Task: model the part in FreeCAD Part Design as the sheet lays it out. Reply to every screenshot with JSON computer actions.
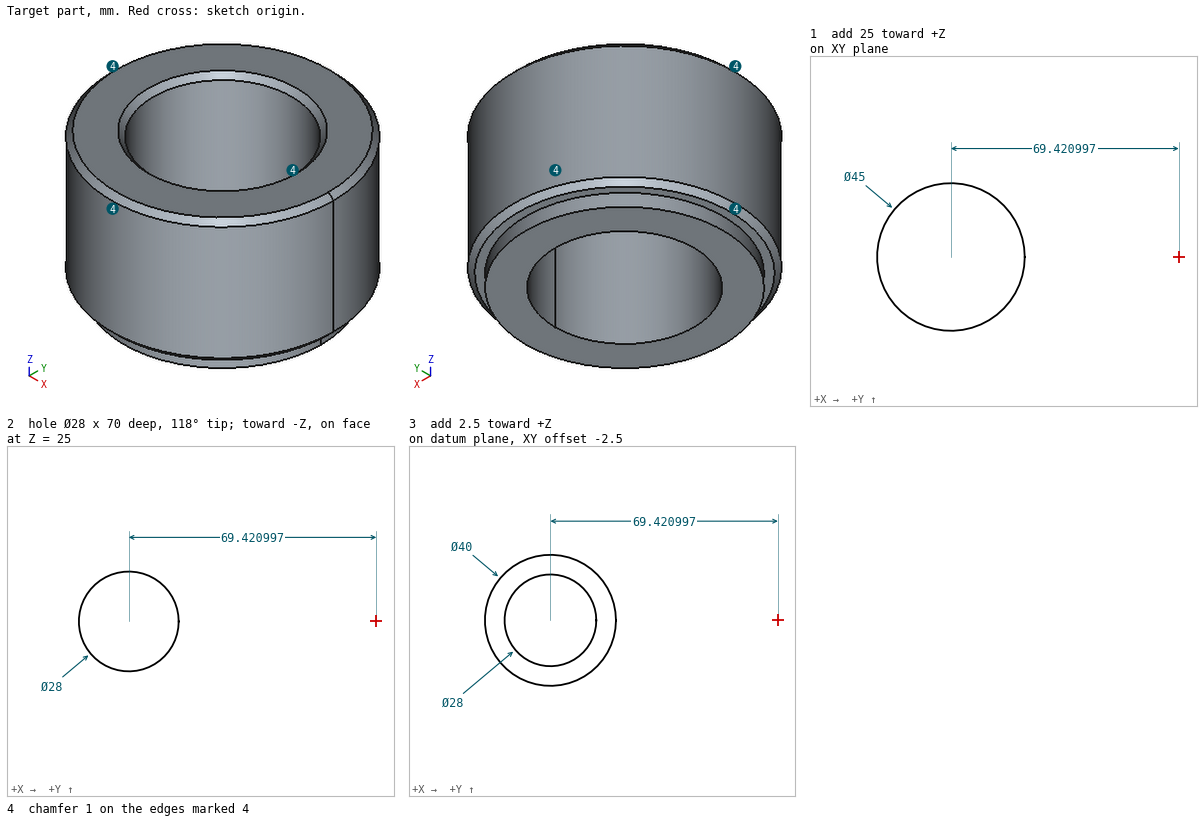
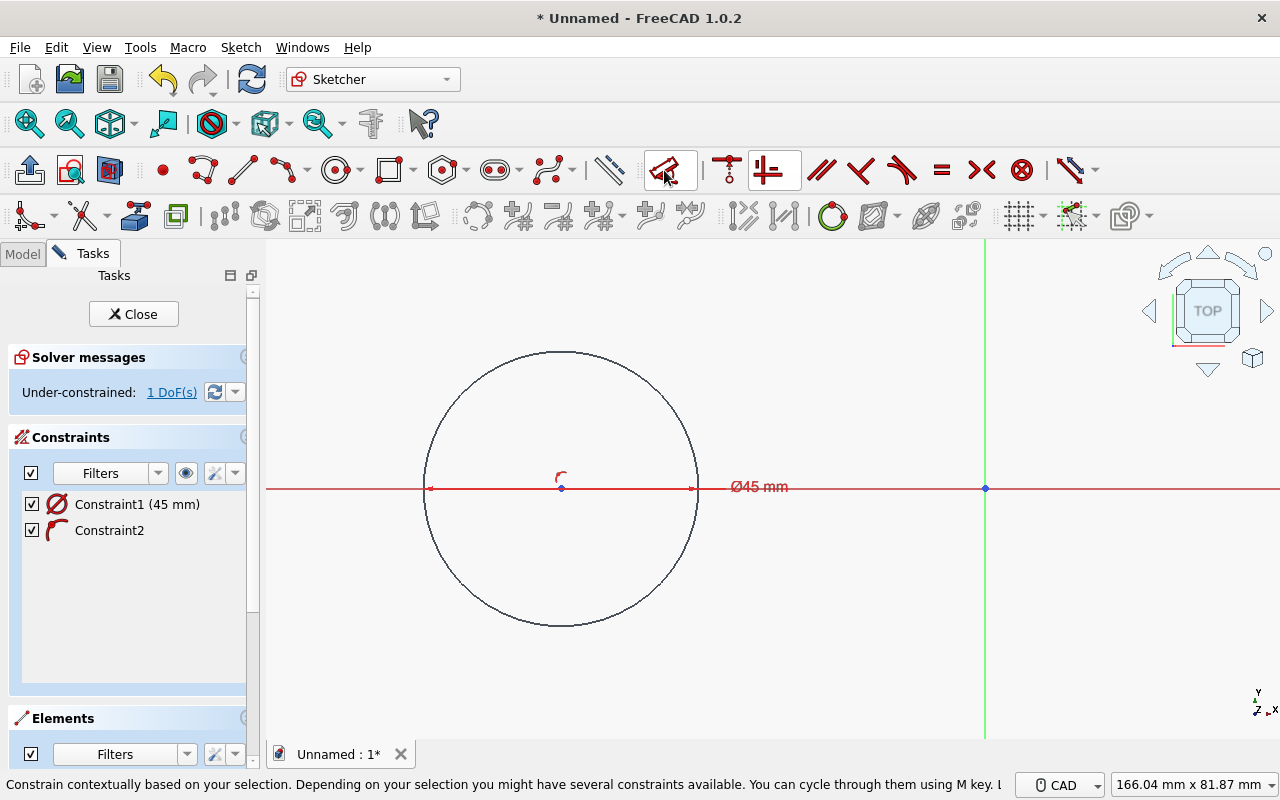
{"action": "left_click", "coordinate": [561, 489]}
{"action": "left_click", "coordinate": [773, 523]}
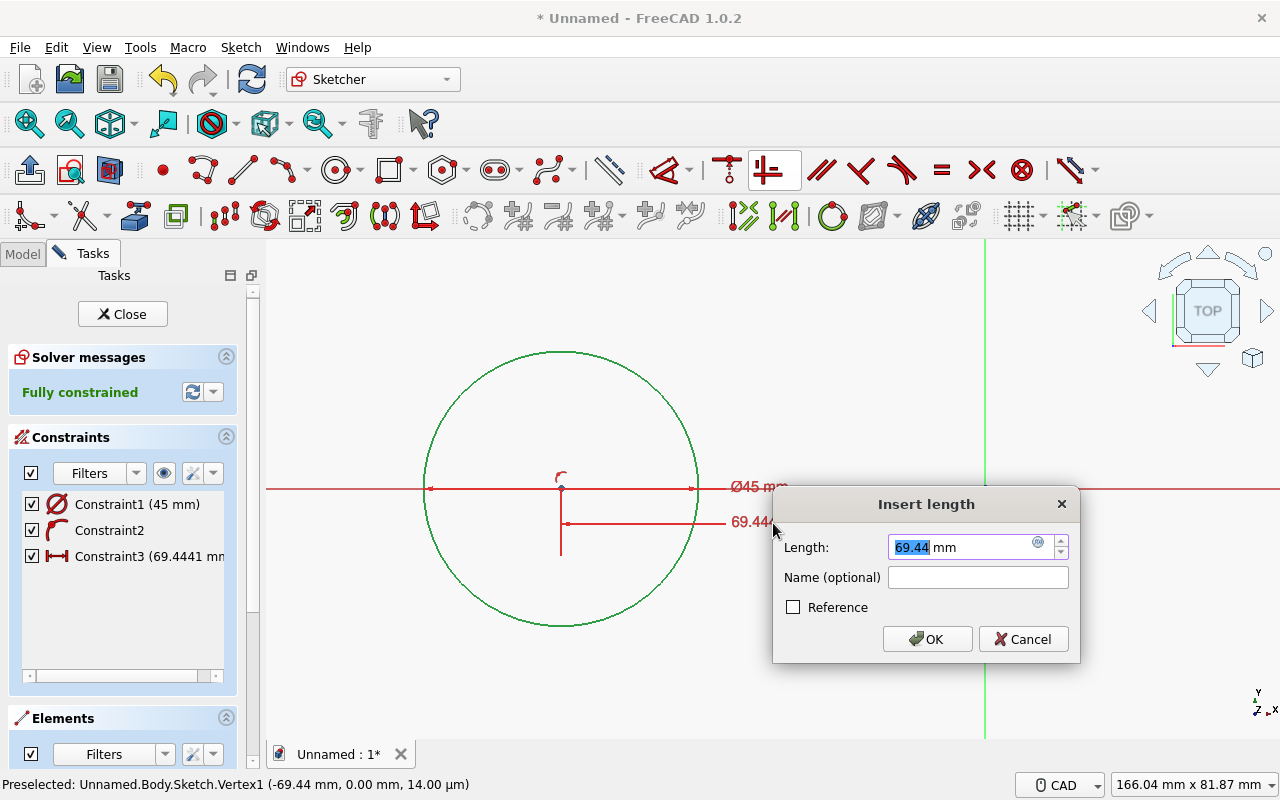
{"action": "type", "text": "69.420997"}
{"action": "key", "text": "Return"}
{"action": "key", "text": "Escape"}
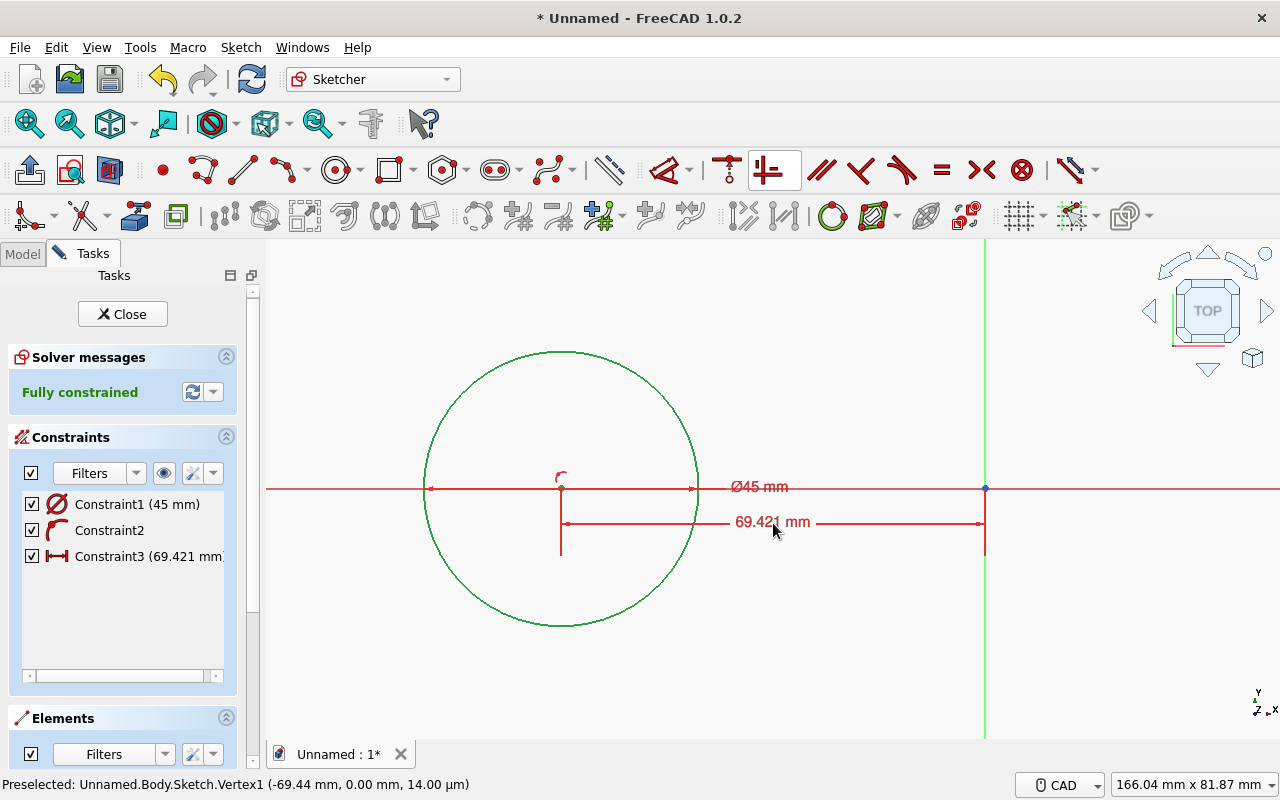
{"action": "left_click", "coordinate": [123, 314]}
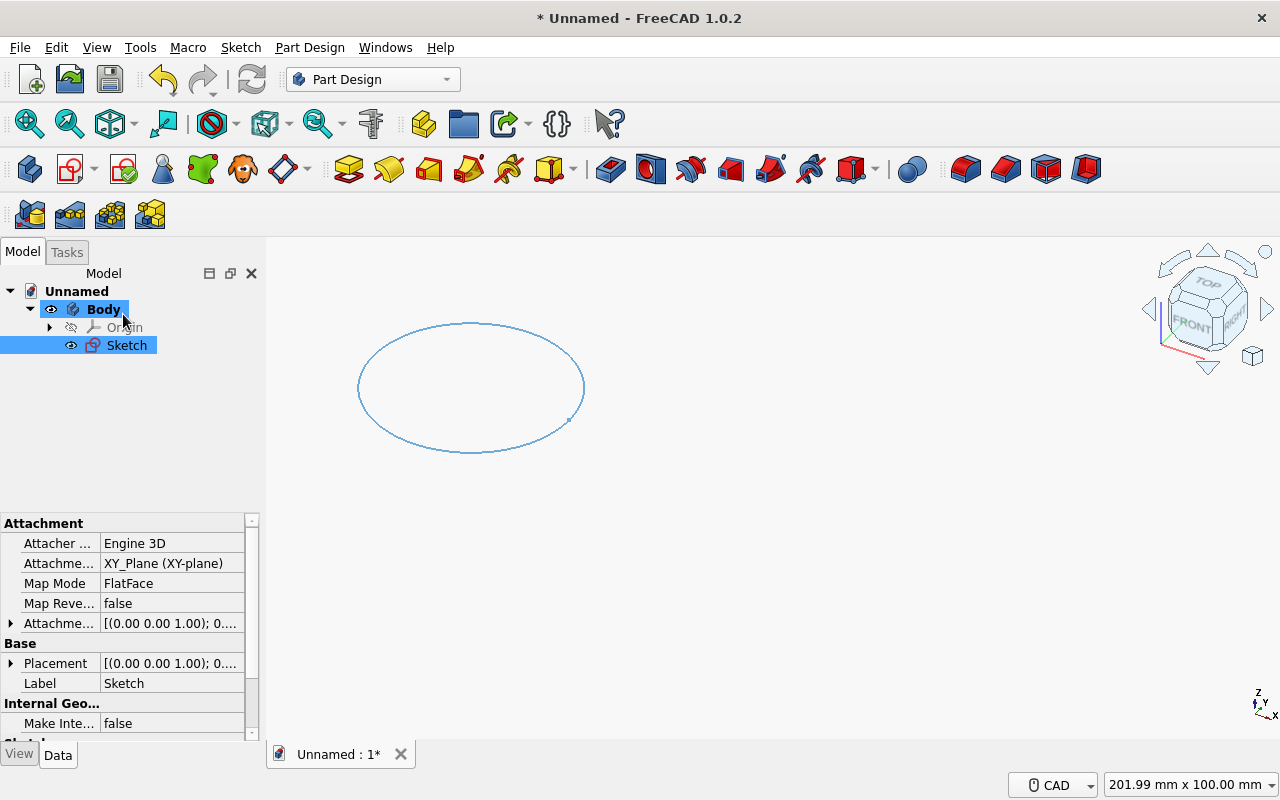
{"action": "left_click", "coordinate": [350, 170]}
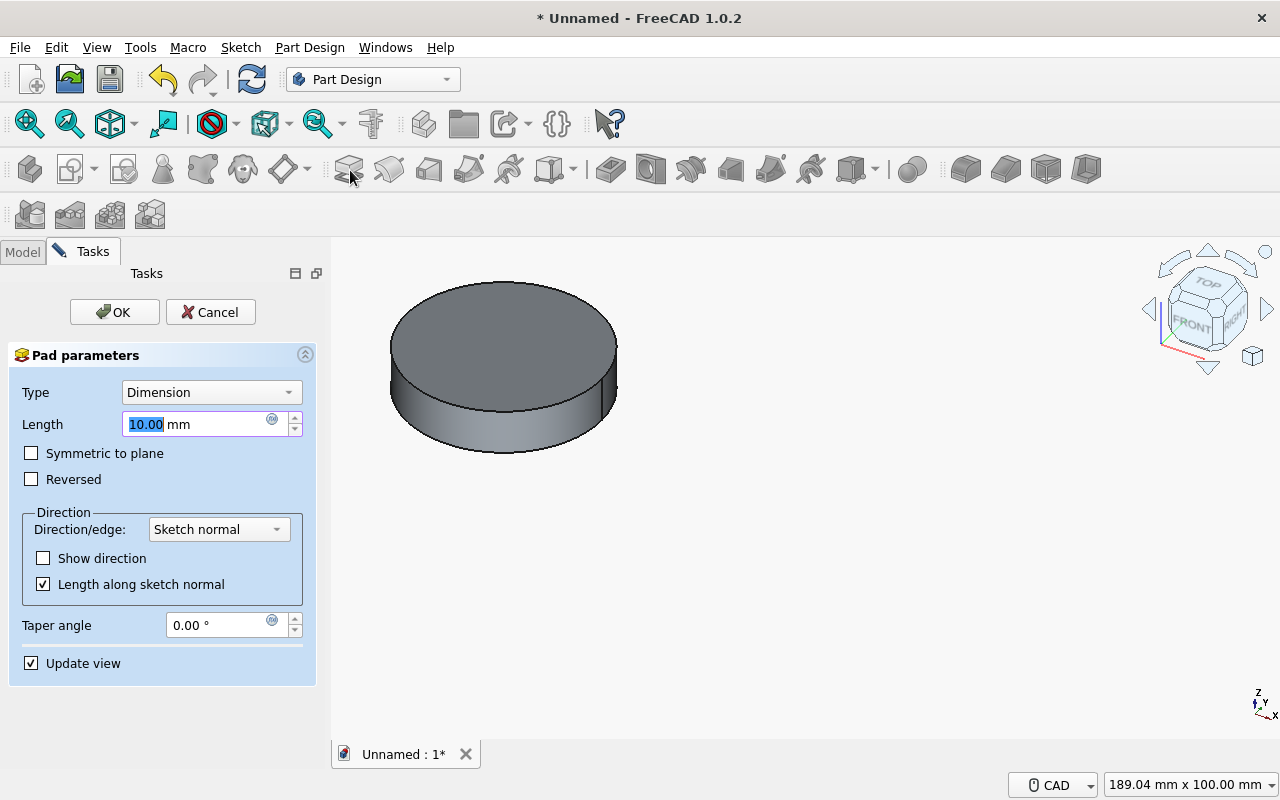
{"action": "type", "text": "25"}
{"action": "key", "text": "Tab"}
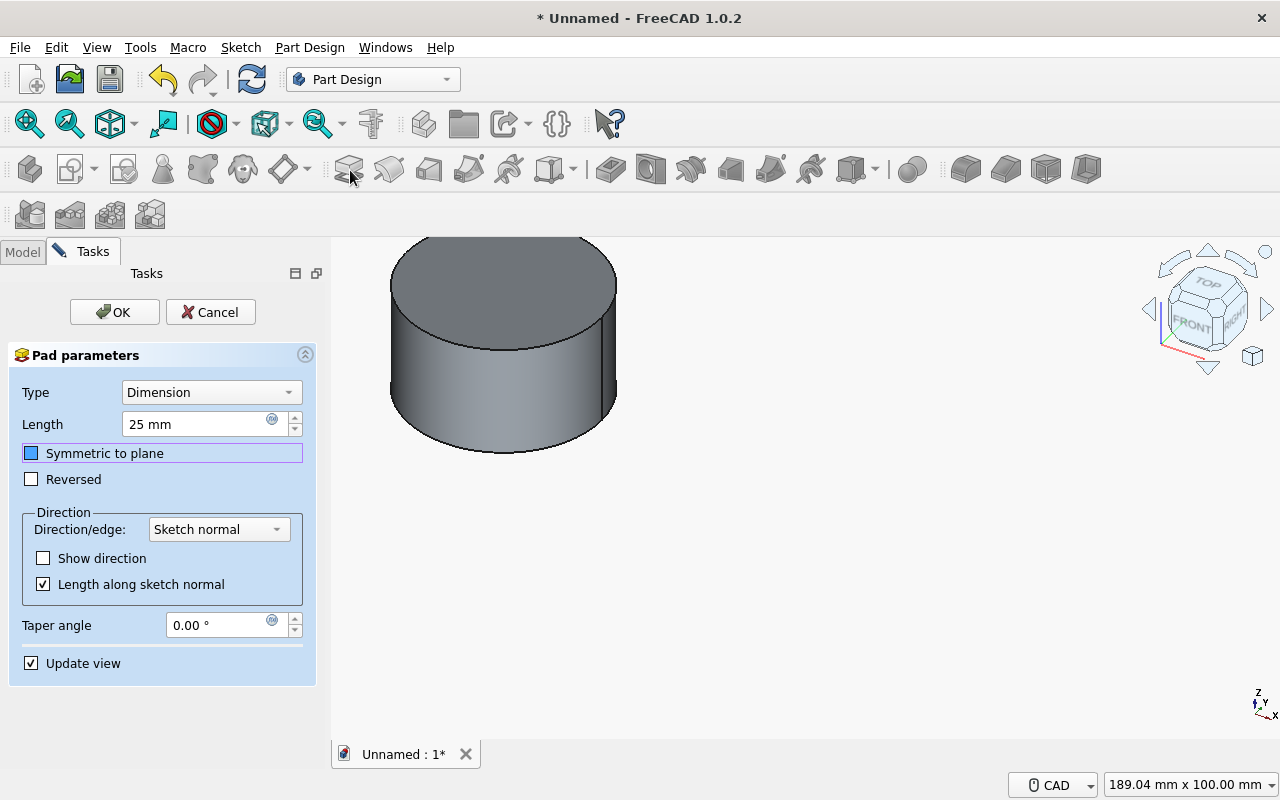
{"action": "left_click", "coordinate": [115, 312]}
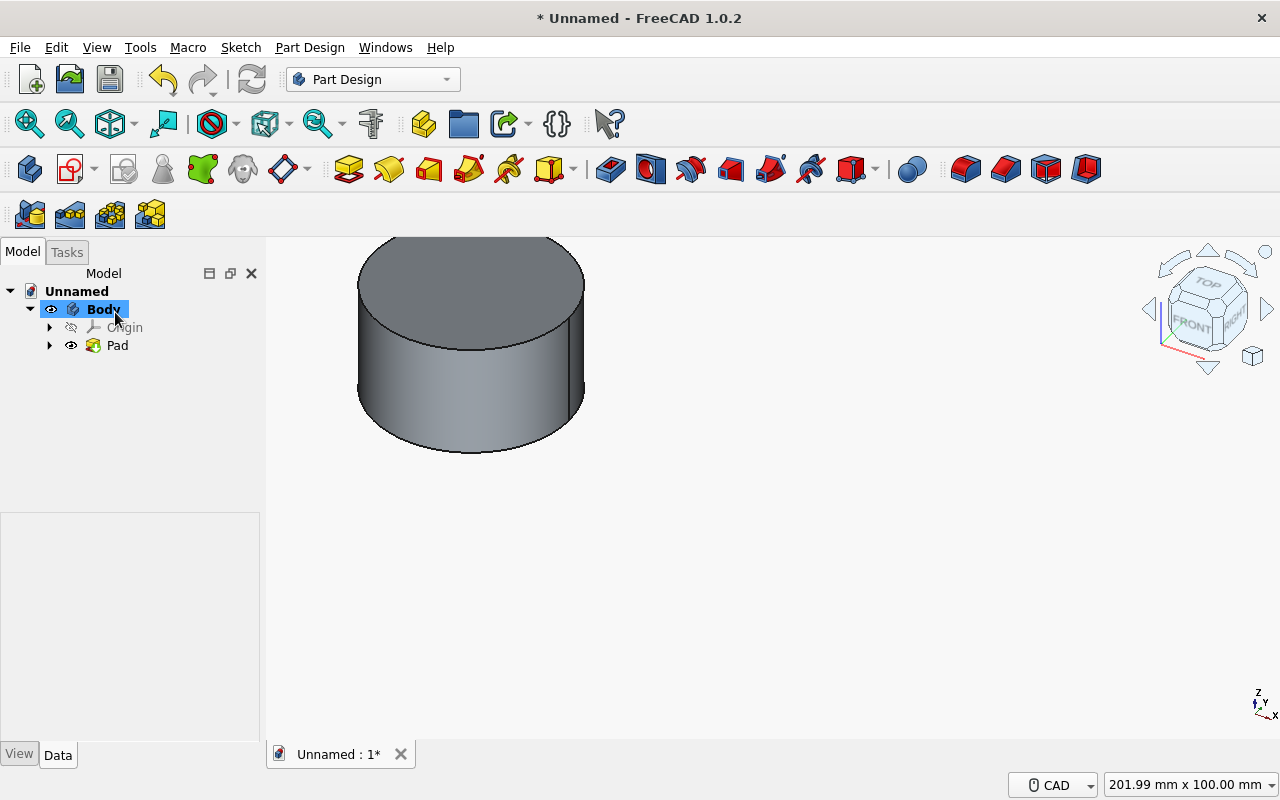
{"action": "key", "text": "v f"}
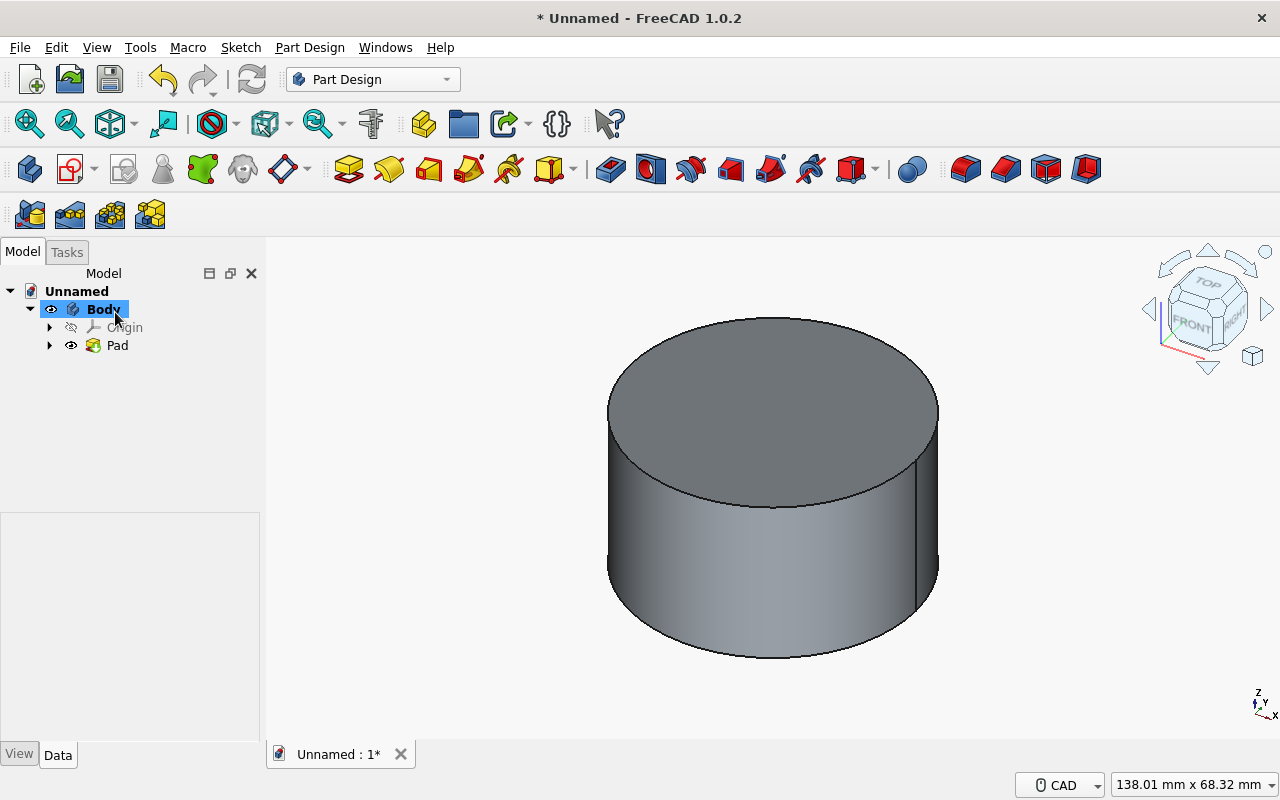
{"action": "left_click", "coordinate": [773, 412]}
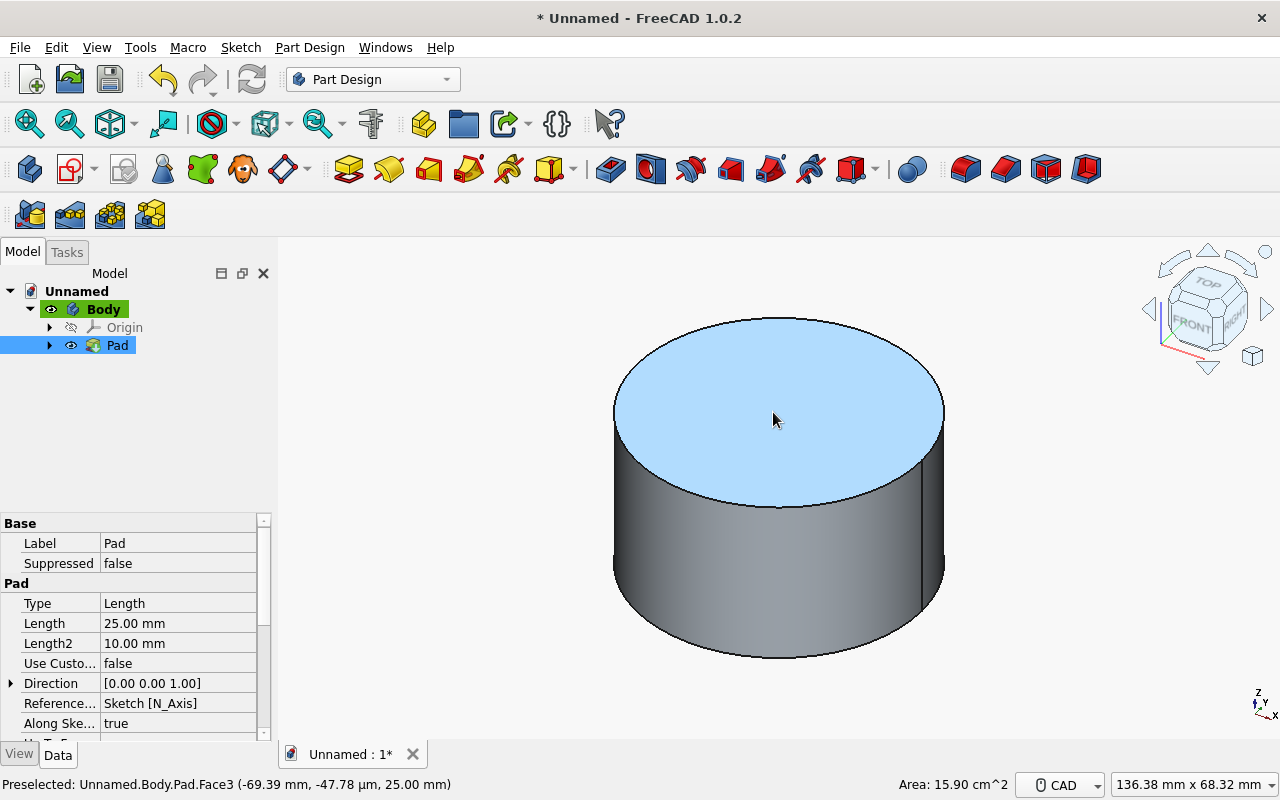
{"action": "left_click", "coordinate": [70, 170]}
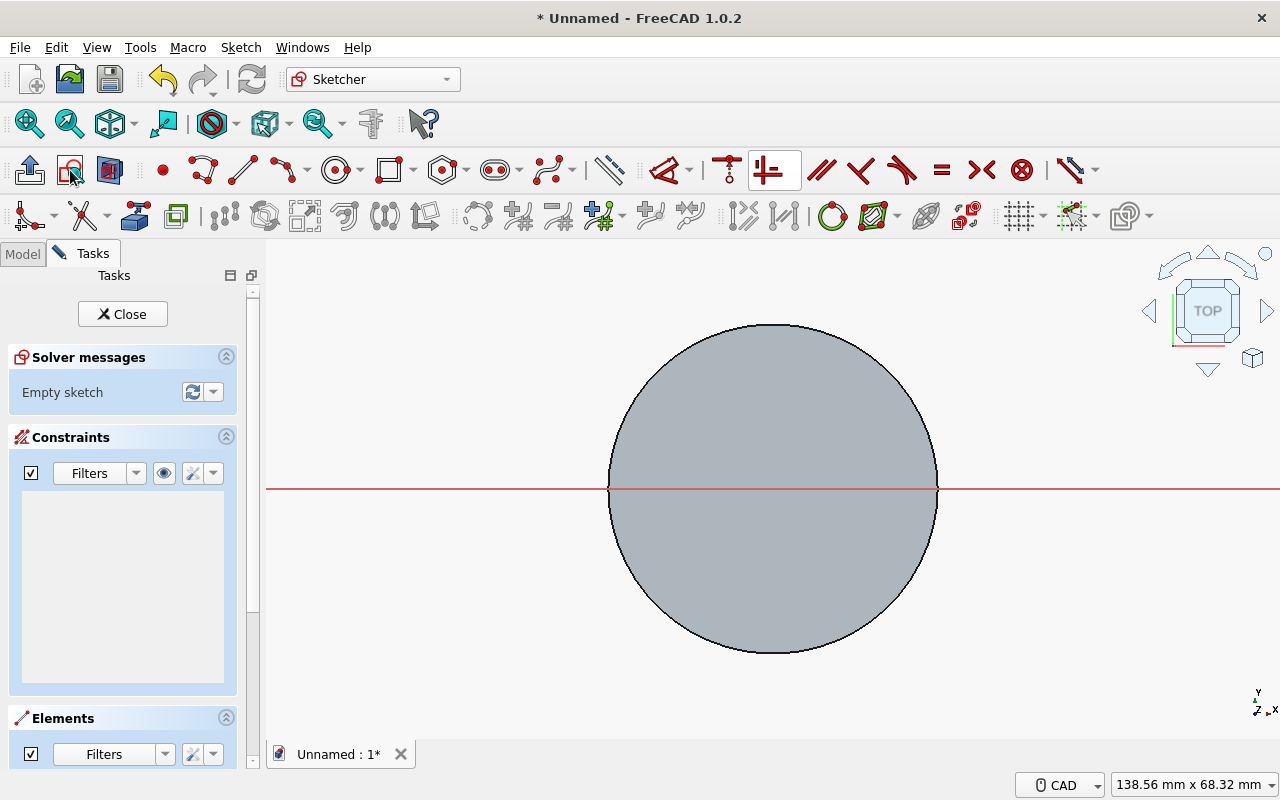
{"action": "scroll", "coordinate": [912, 489], "scroll_direction": "up", "scroll_amount": 2}